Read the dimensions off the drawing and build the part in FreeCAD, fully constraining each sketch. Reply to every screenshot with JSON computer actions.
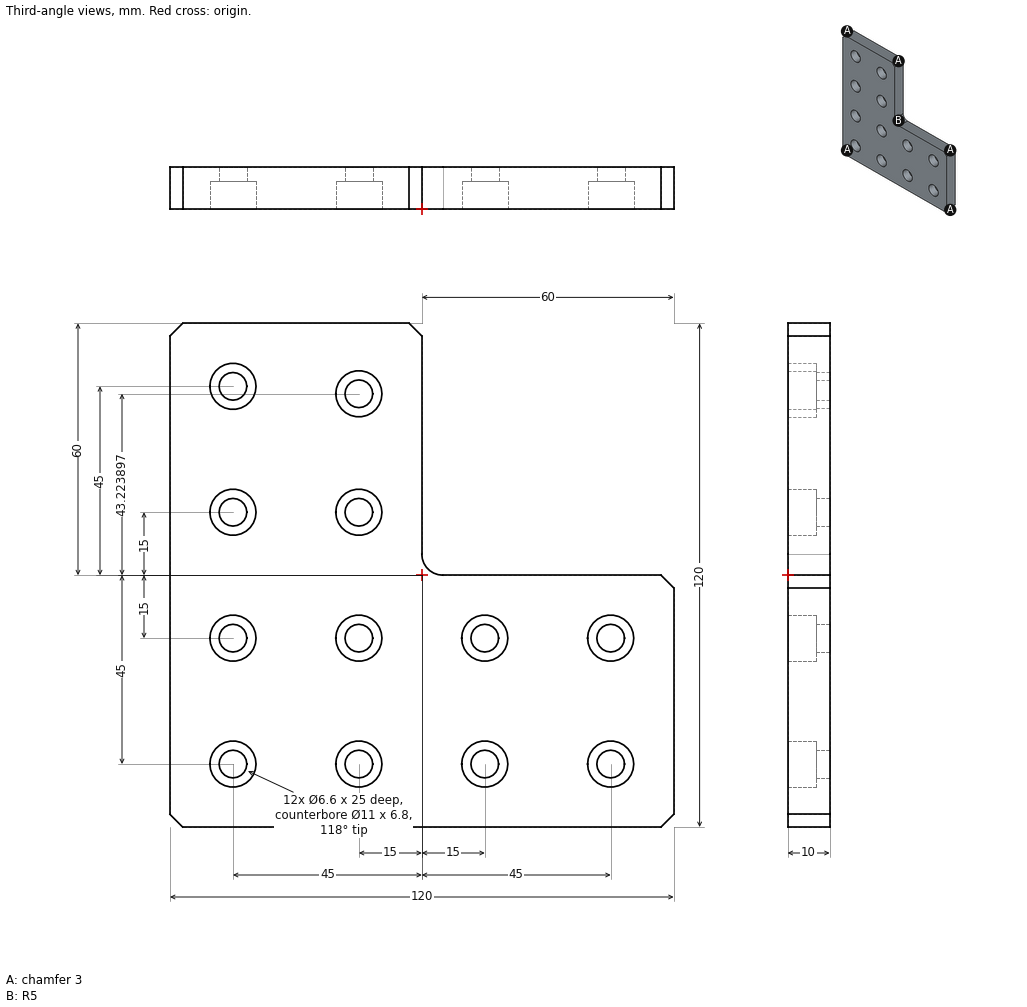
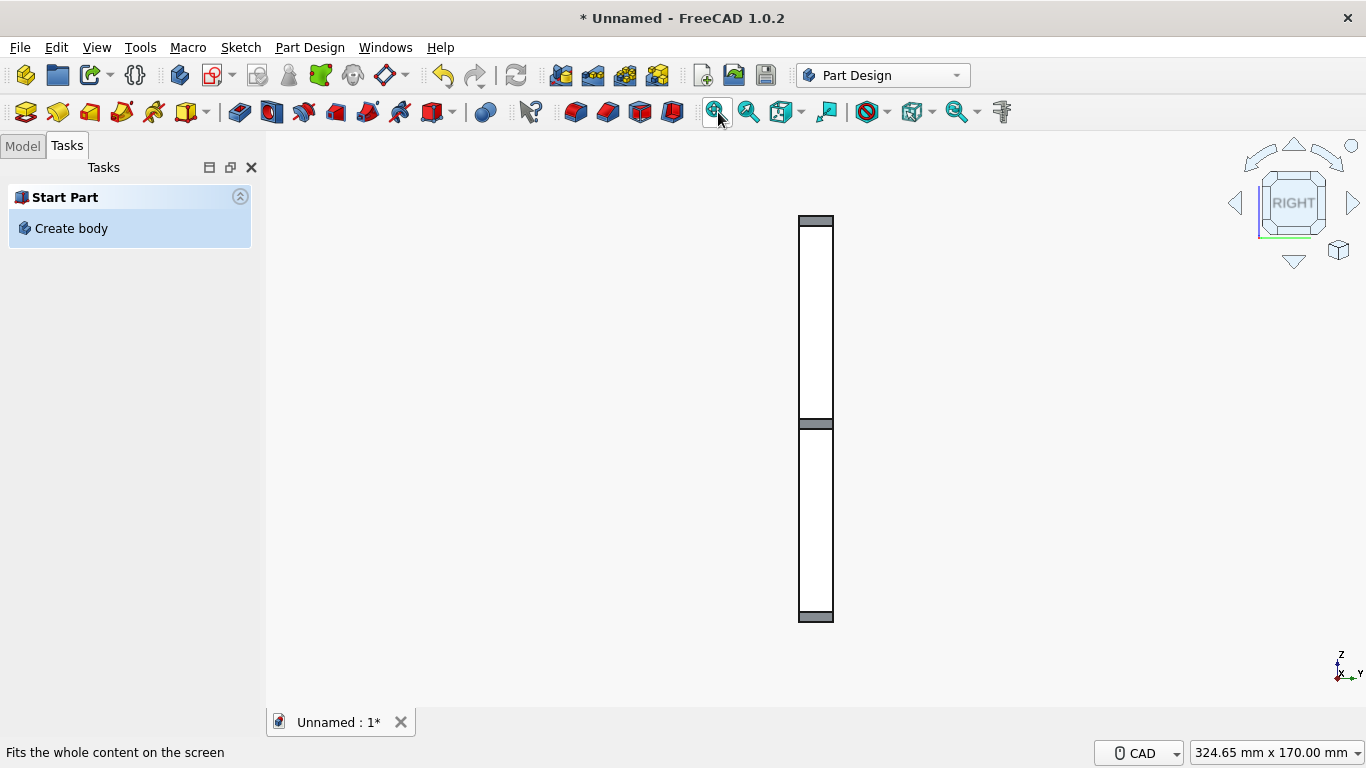
{"action": "key", "text": "5"}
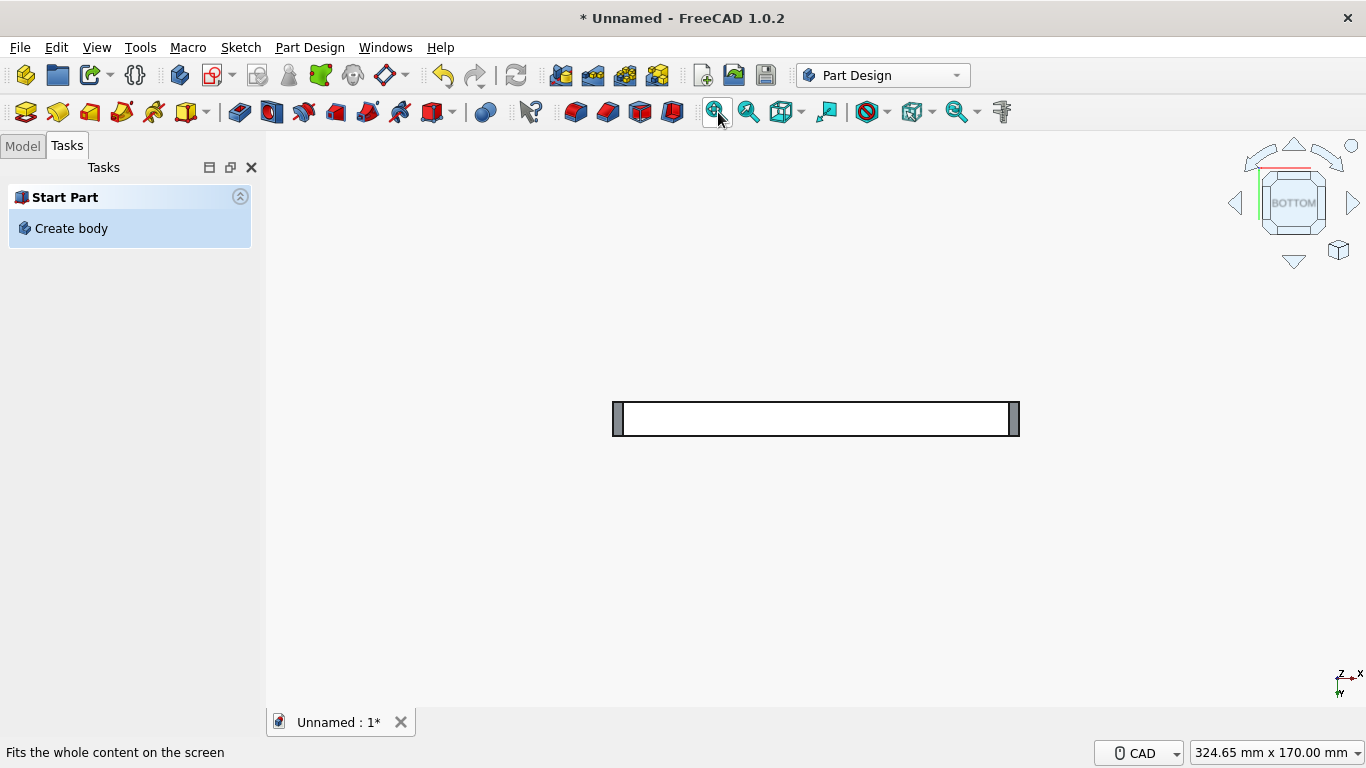
{"action": "left_click", "coordinate": [718, 112]}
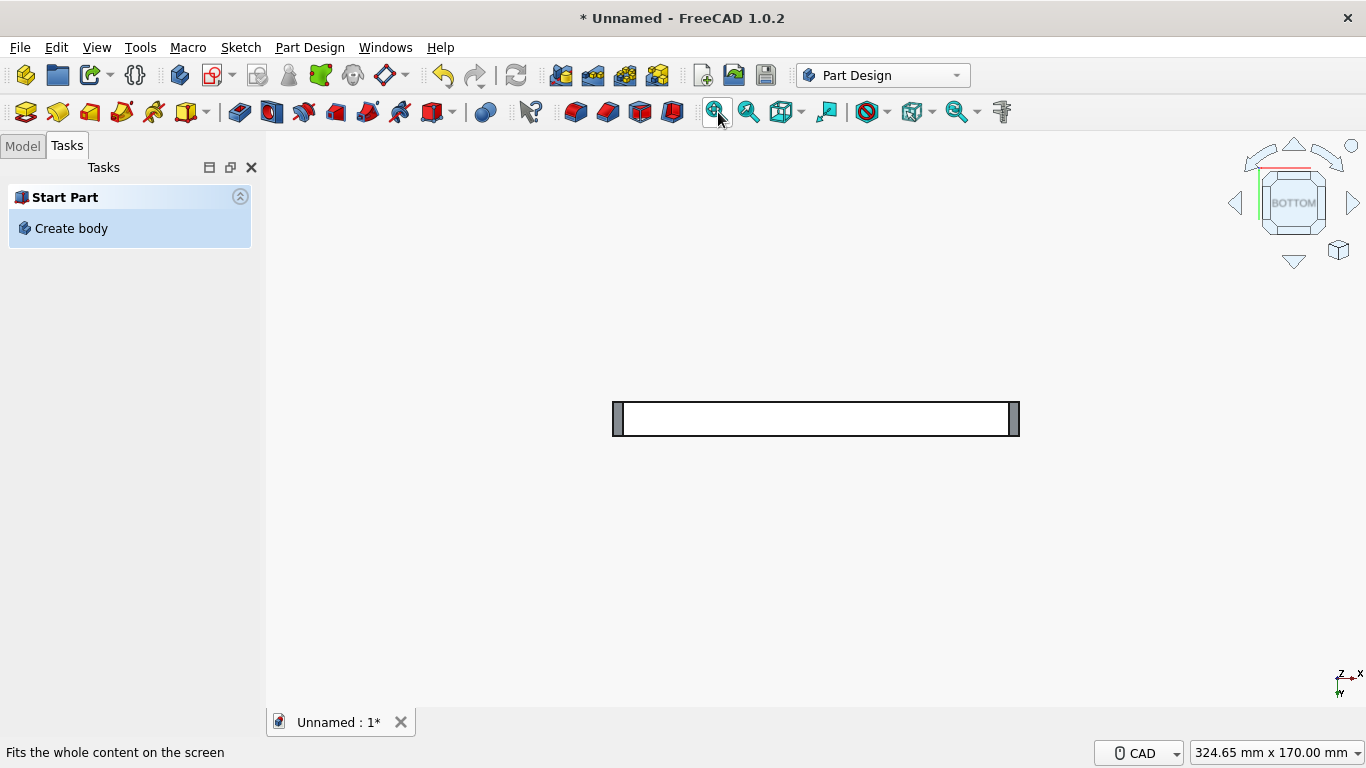
{"action": "key", "text": "4"}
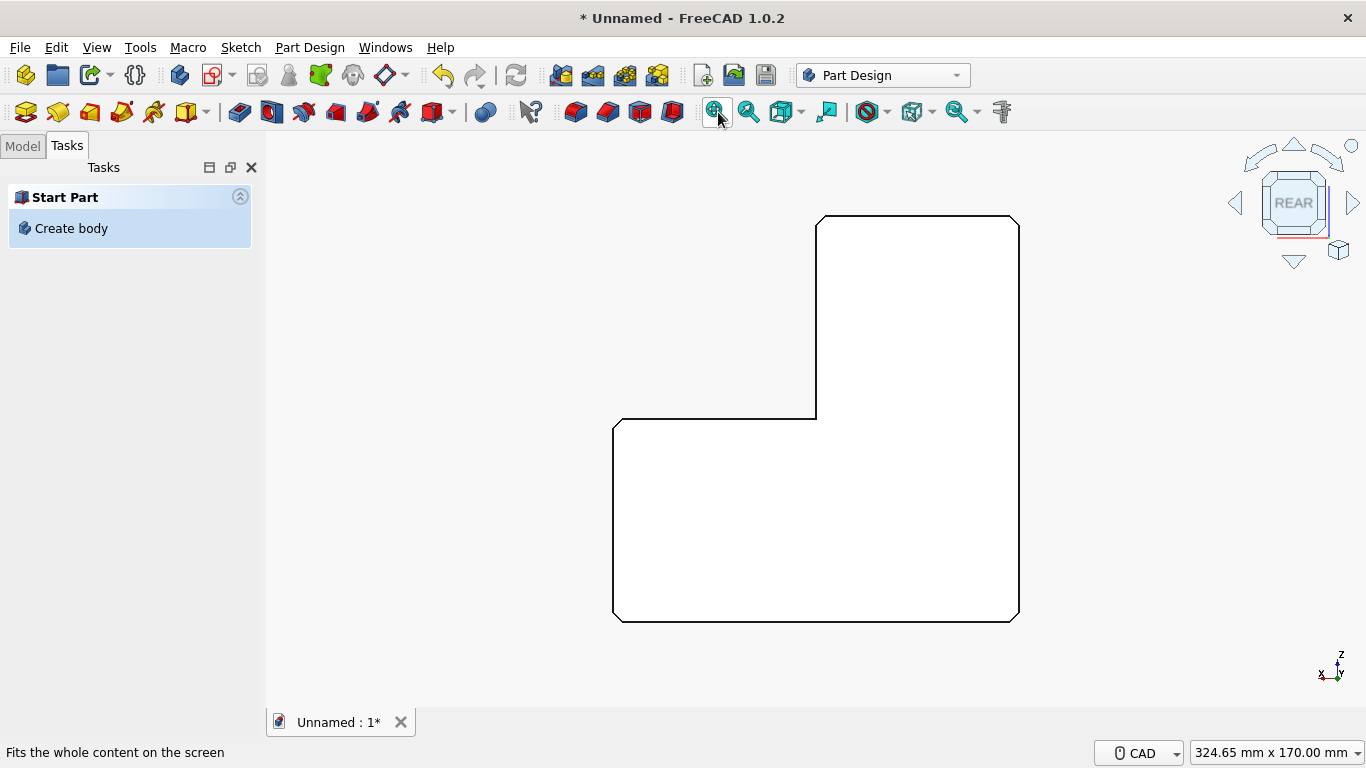
{"action": "key", "text": "6"}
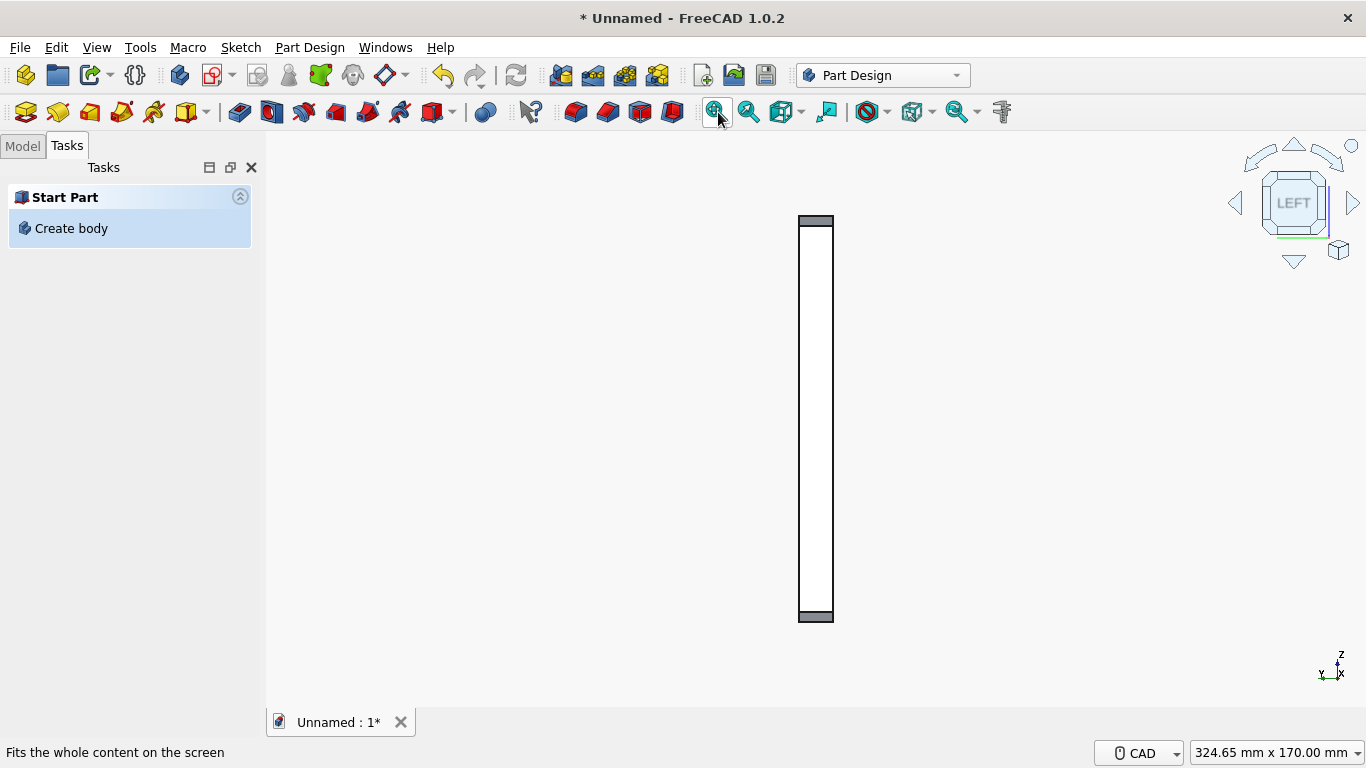
{"action": "key", "text": "v 3"}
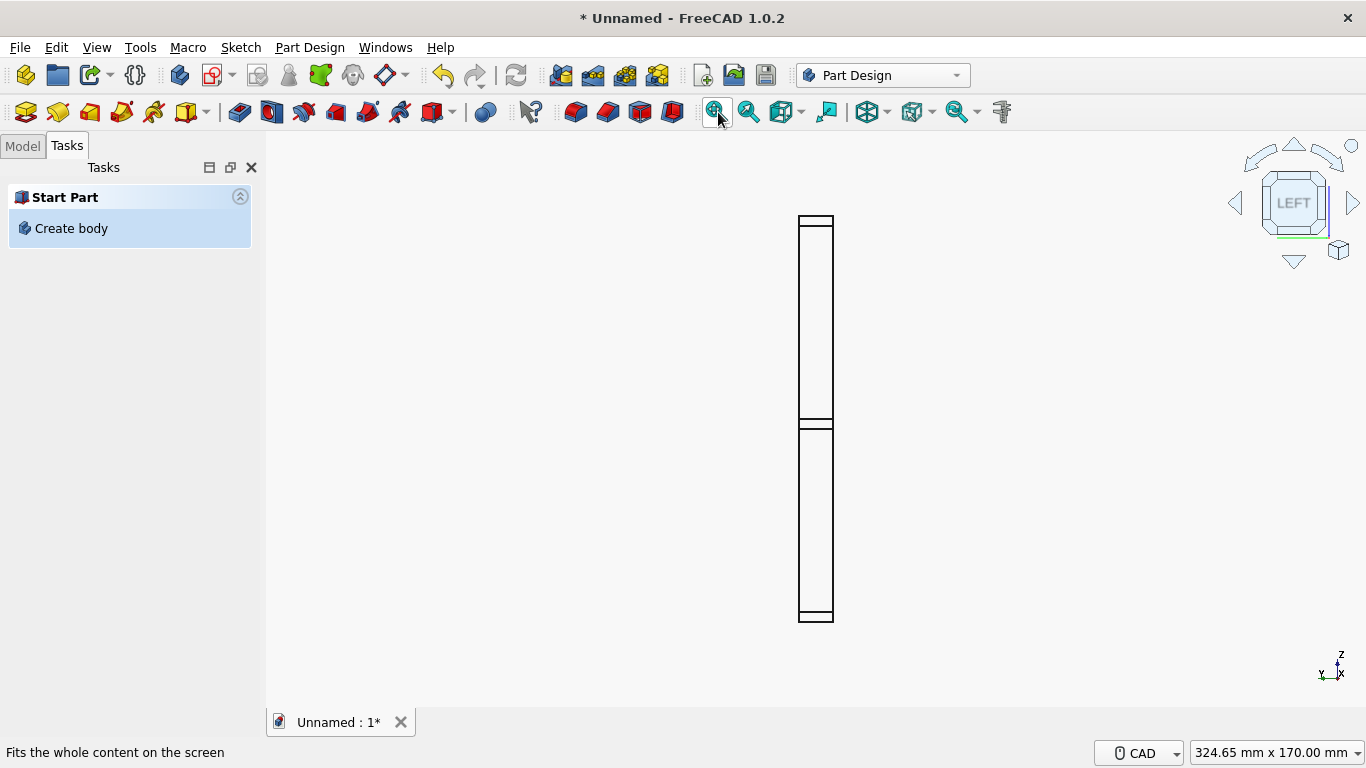
{"action": "key", "text": "0"}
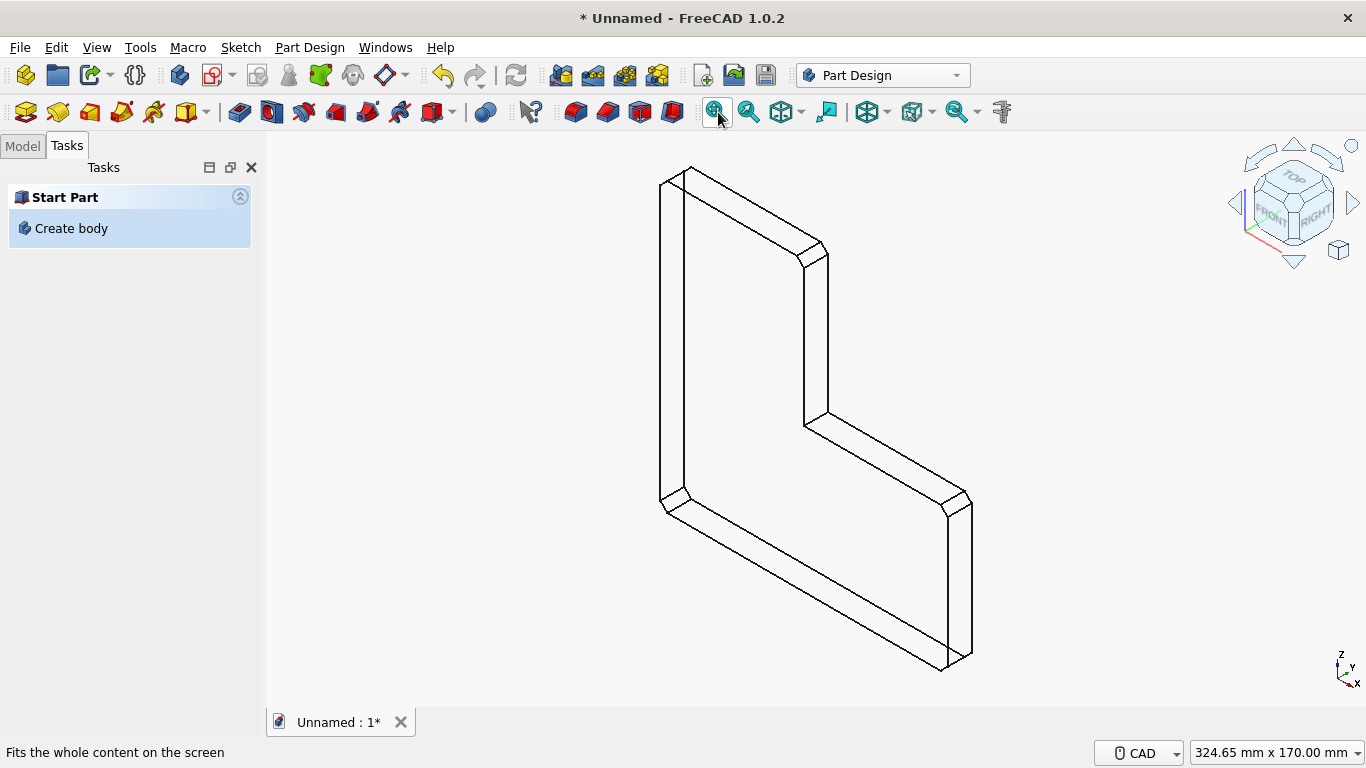
{"action": "left_click", "coordinate": [816, 418]}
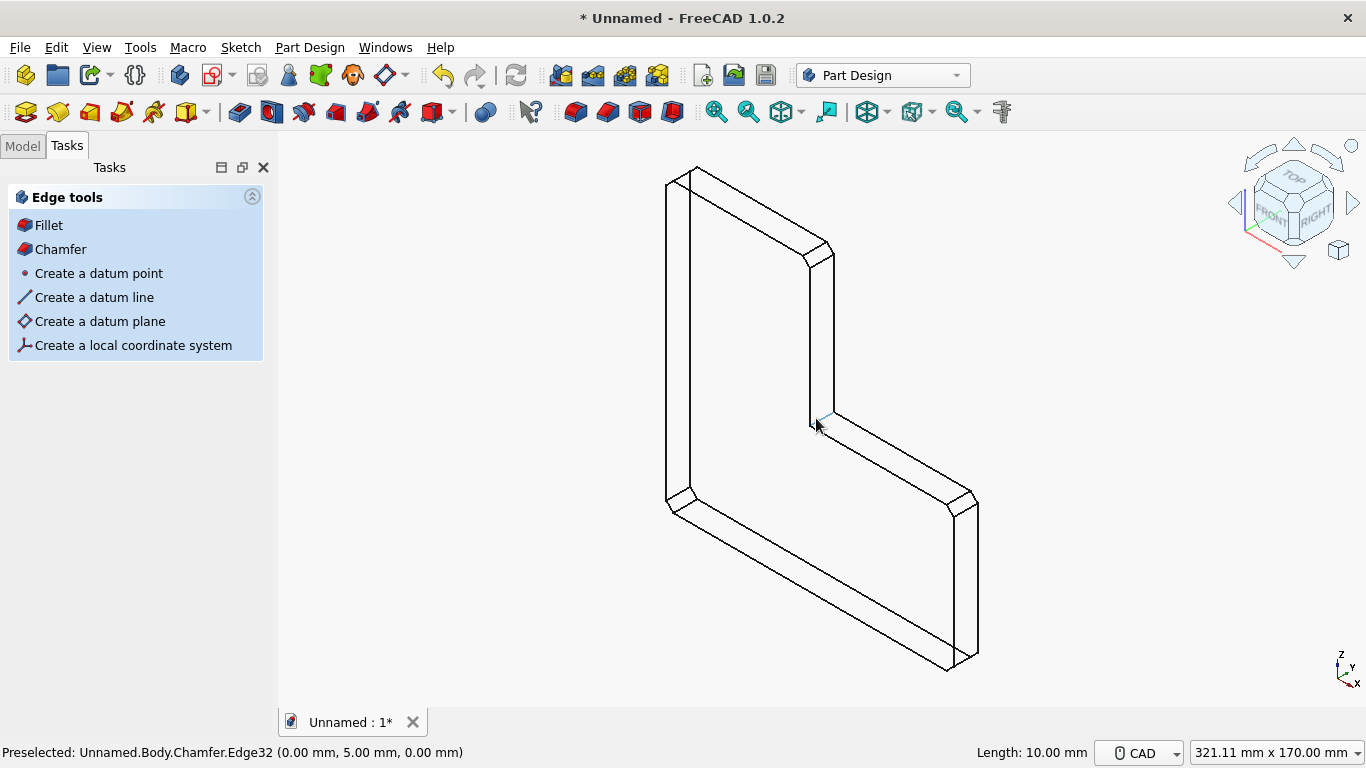
{"action": "key", "text": "v 1"}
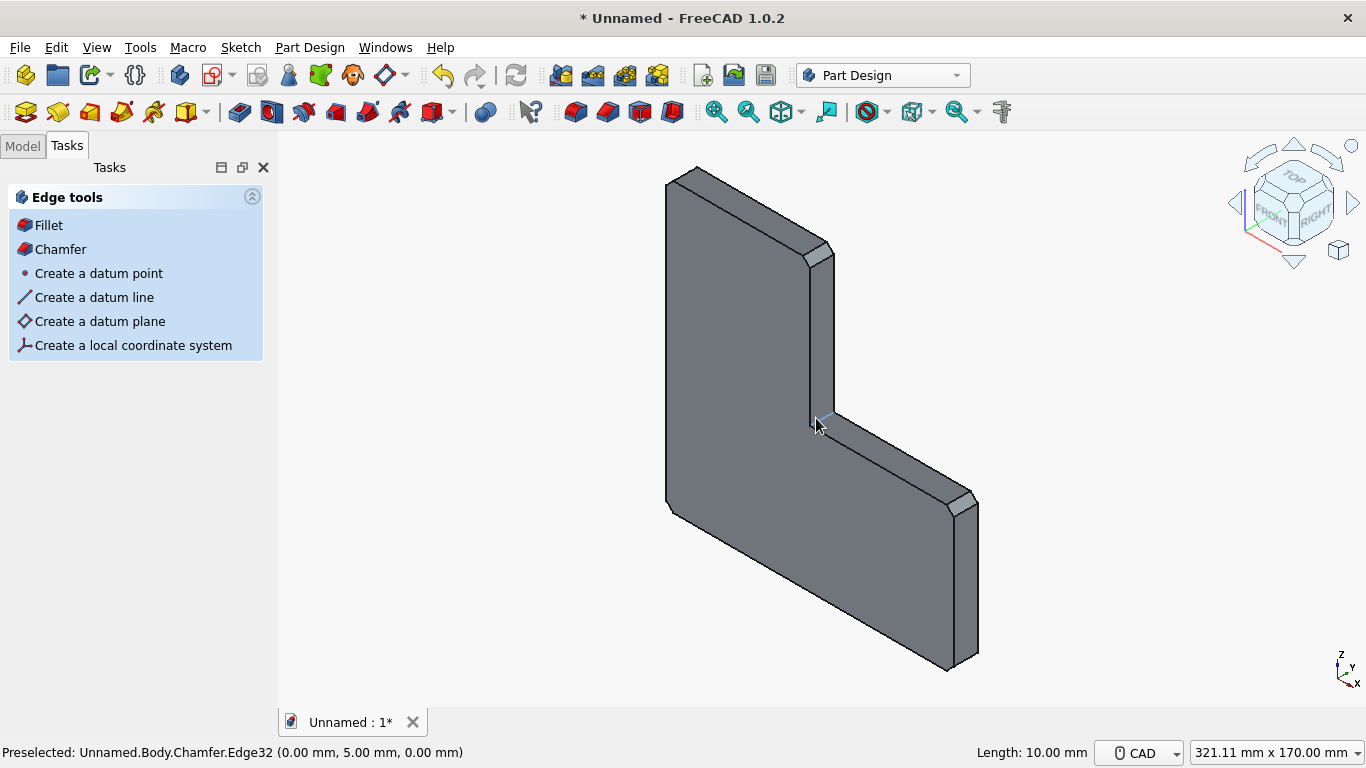
{"action": "left_click", "coordinate": [576, 112]}